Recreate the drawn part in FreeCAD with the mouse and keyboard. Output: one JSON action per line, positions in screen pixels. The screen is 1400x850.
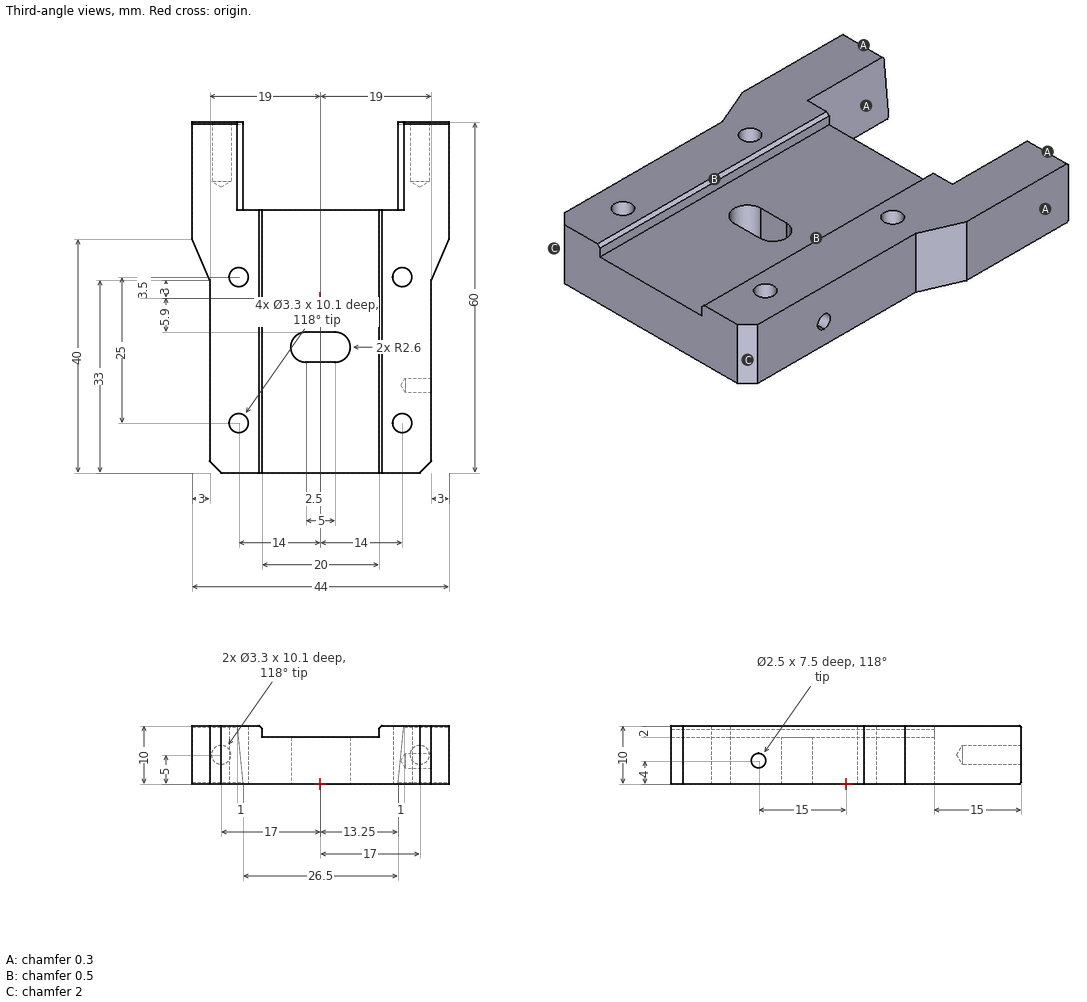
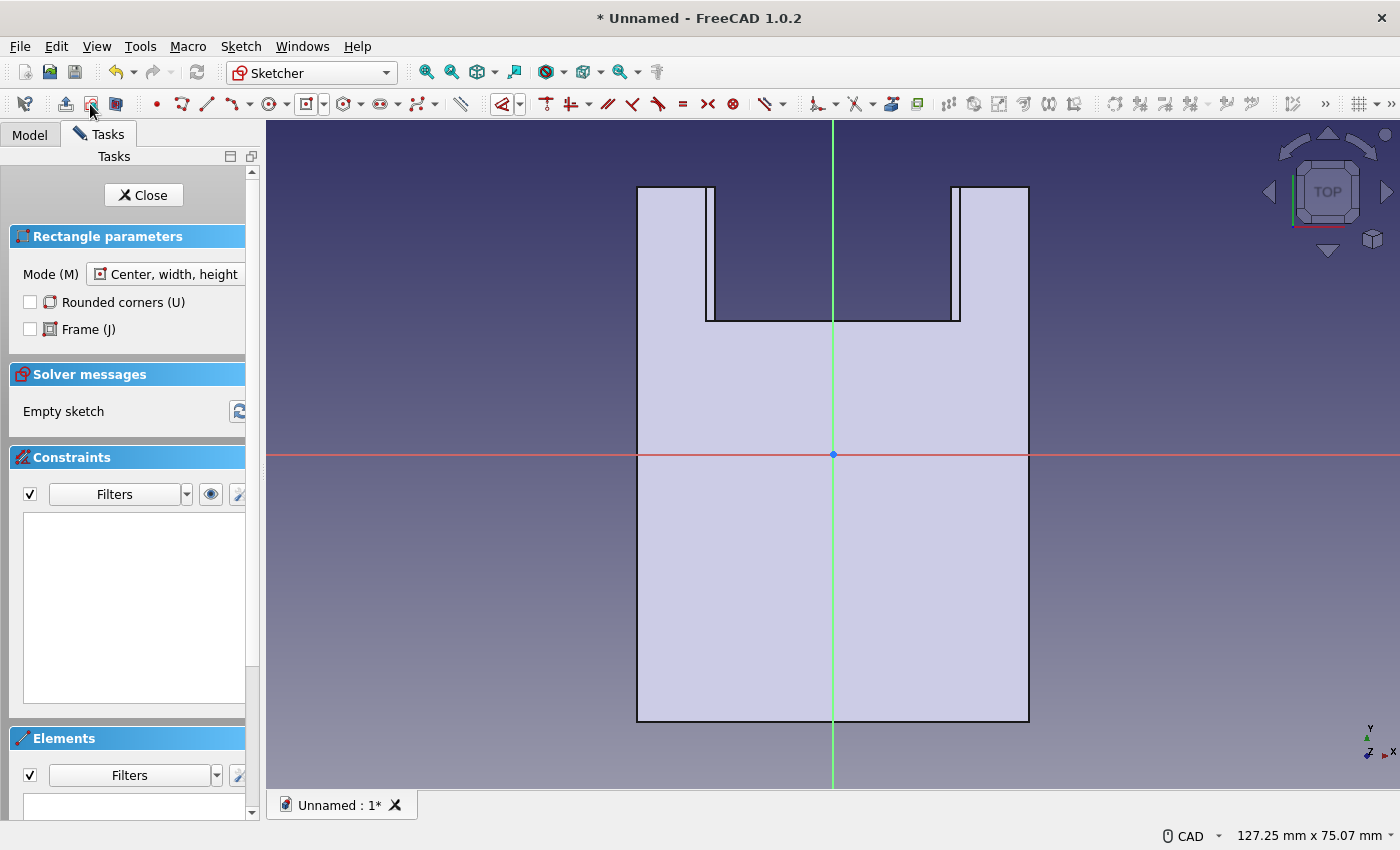
{"action": "left_click", "coordinate": [833, 454]}
{"action": "left_click", "coordinate": [922, 187]}
{"action": "key", "text": "Escape"}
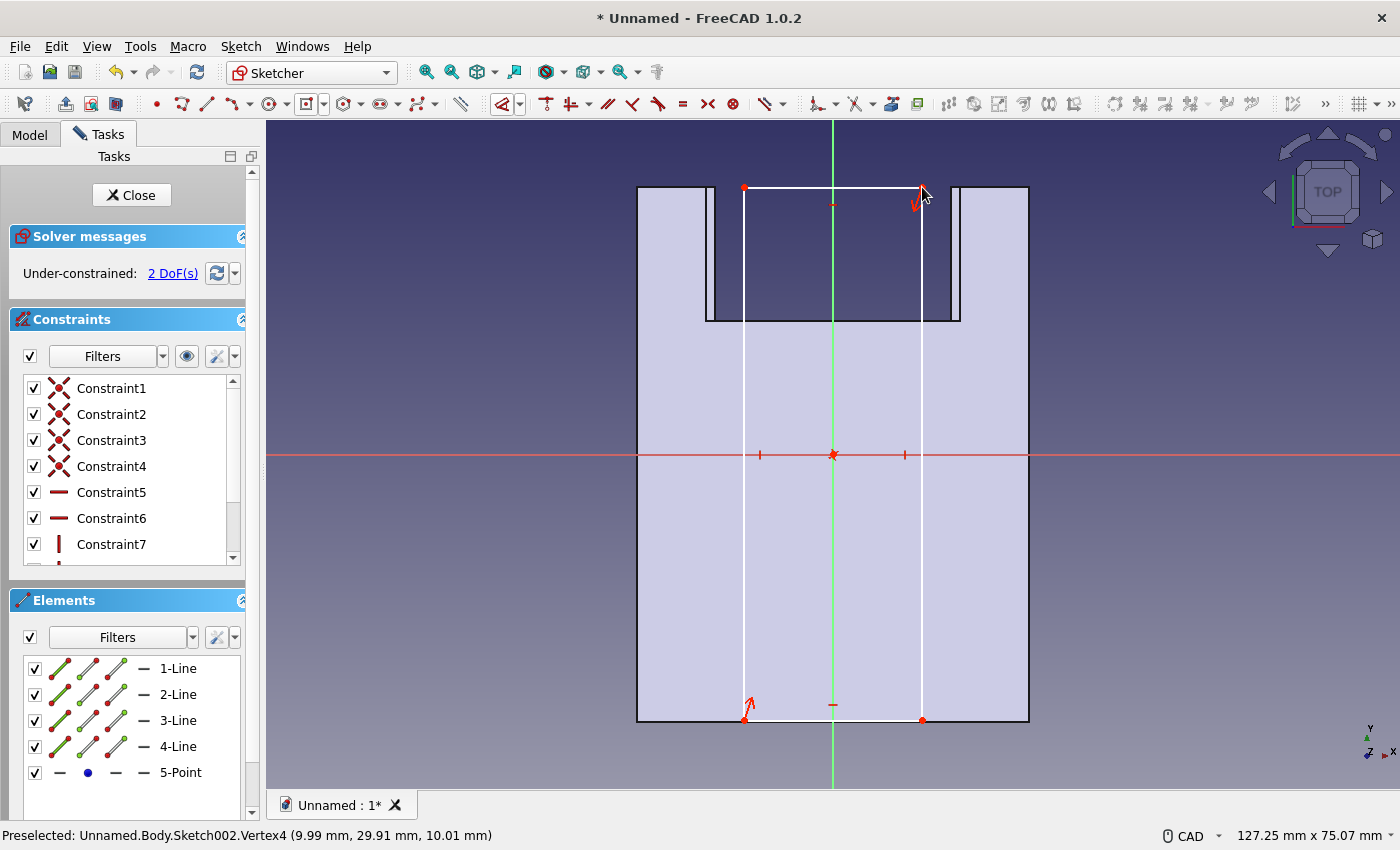
{"action": "left_click", "coordinate": [797, 721]}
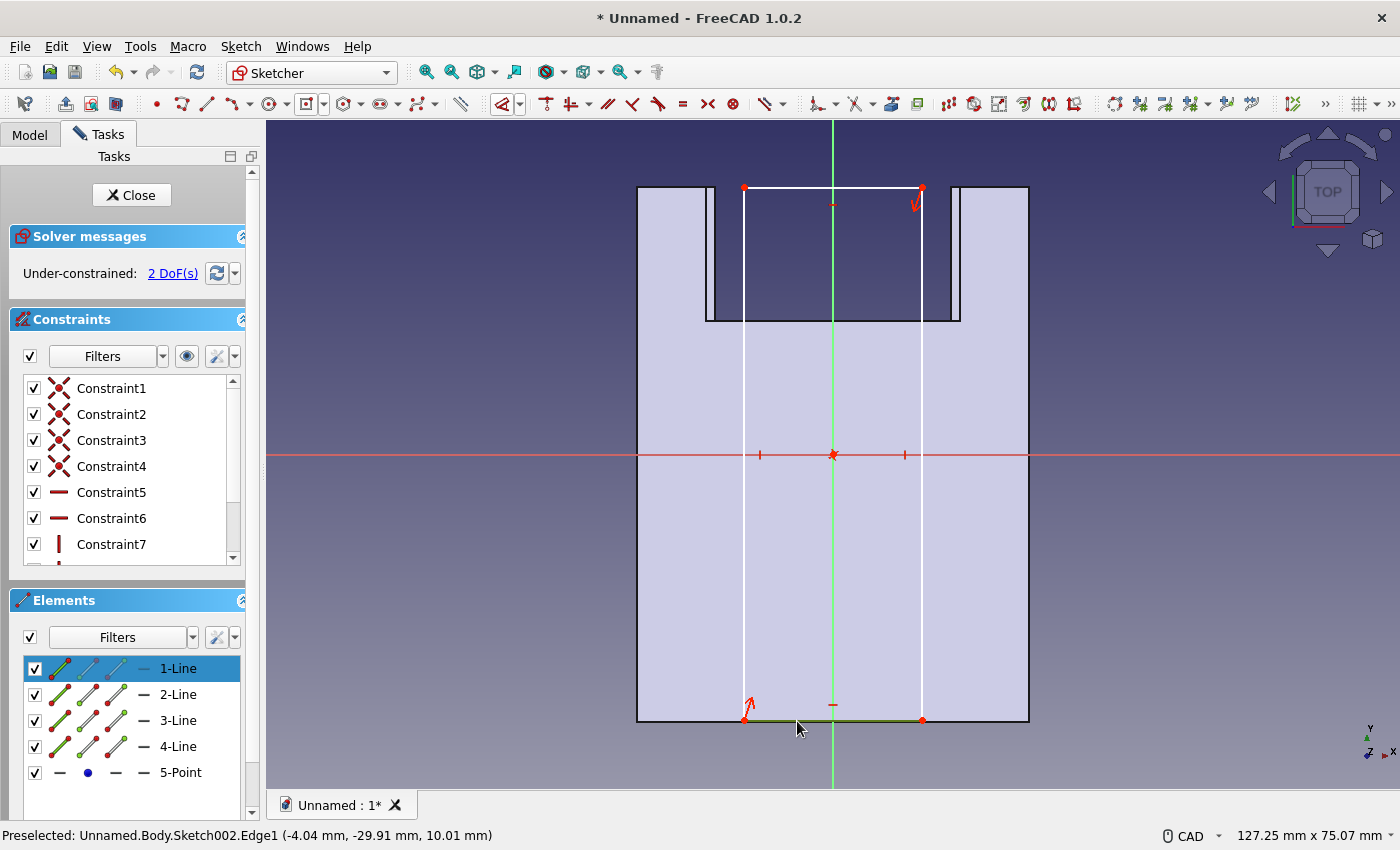
{"action": "key", "text": "l"}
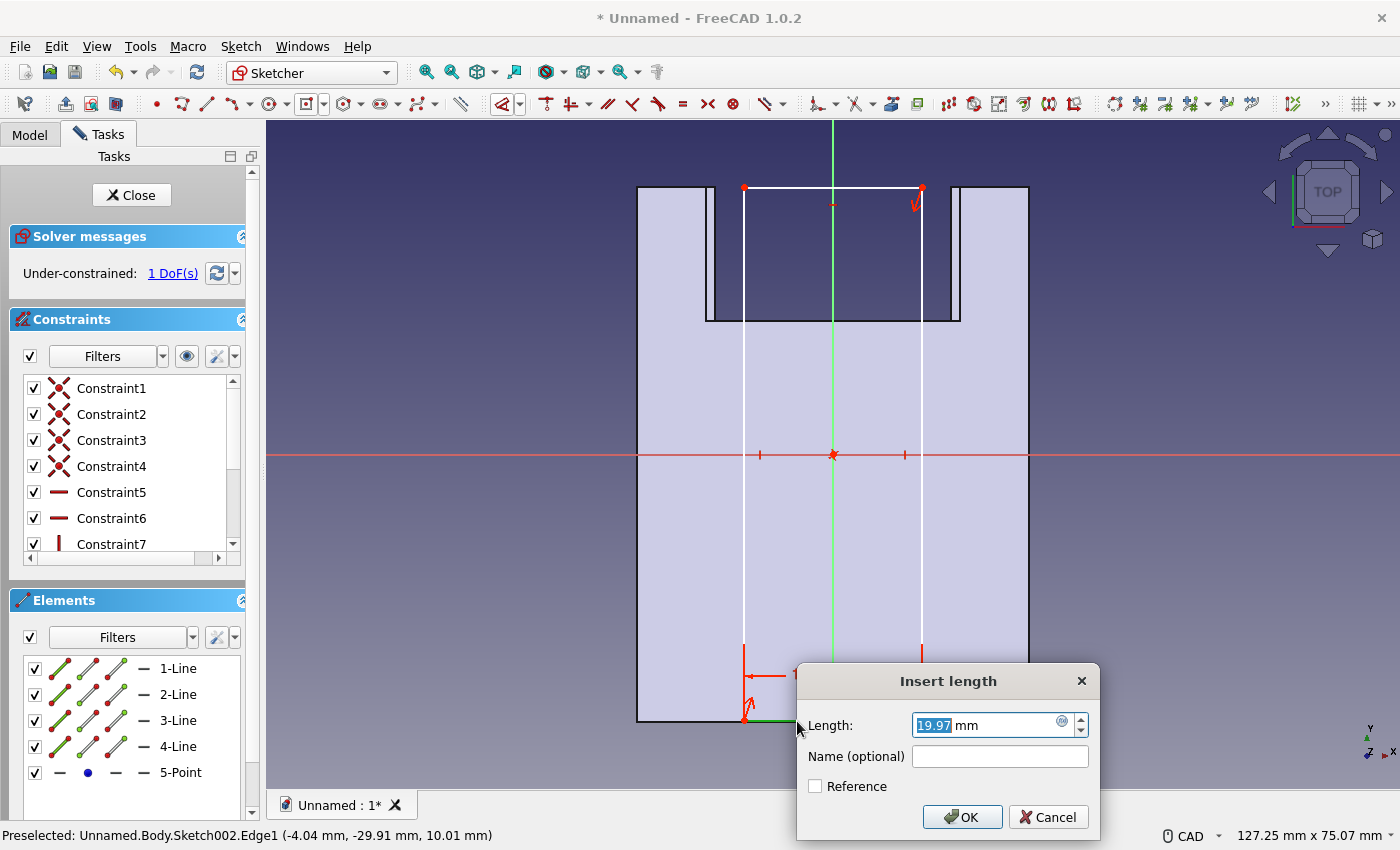
{"action": "type", "text": "20"}
{"action": "key", "text": "Return"}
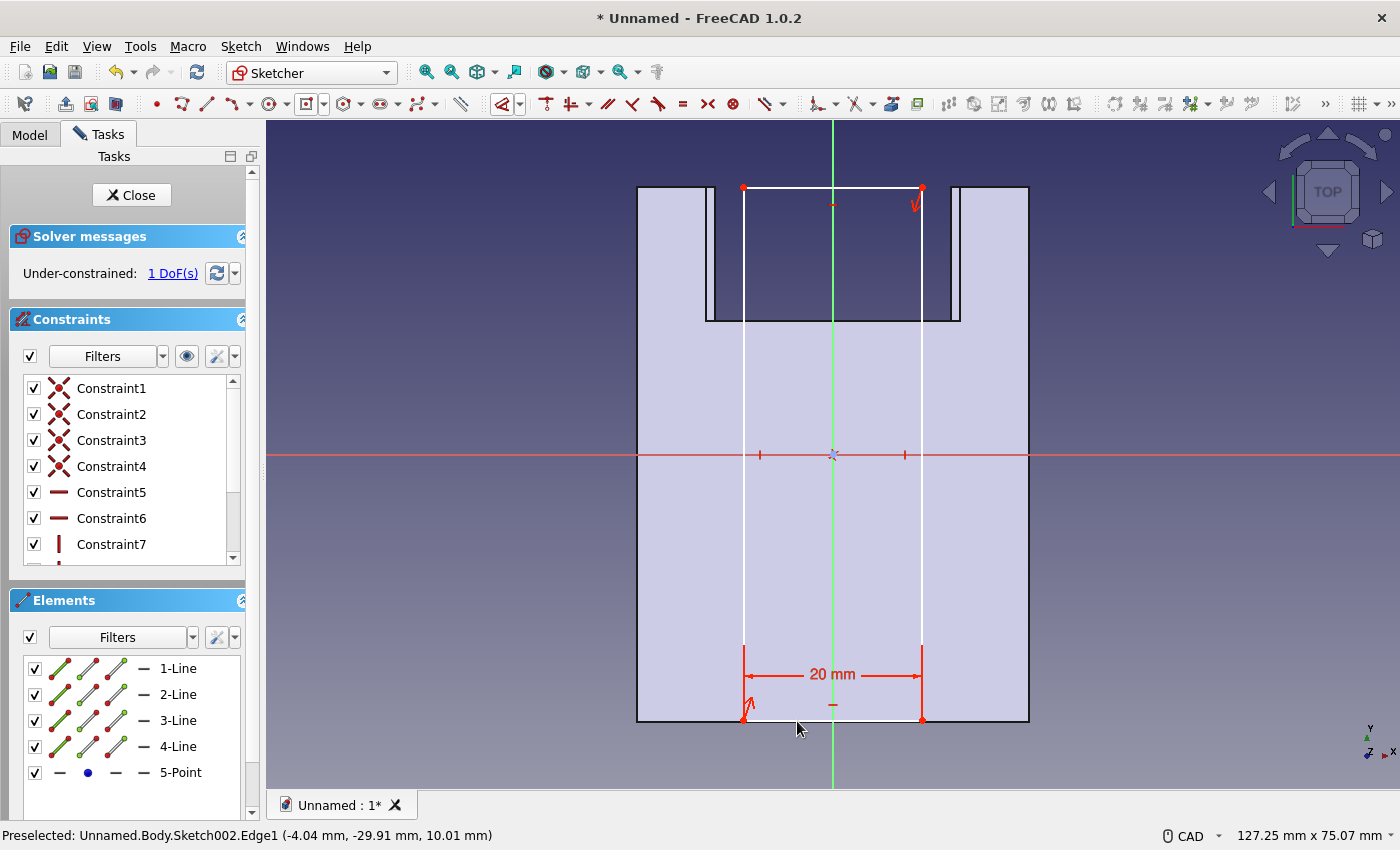
{"action": "left_click", "coordinate": [922, 561]}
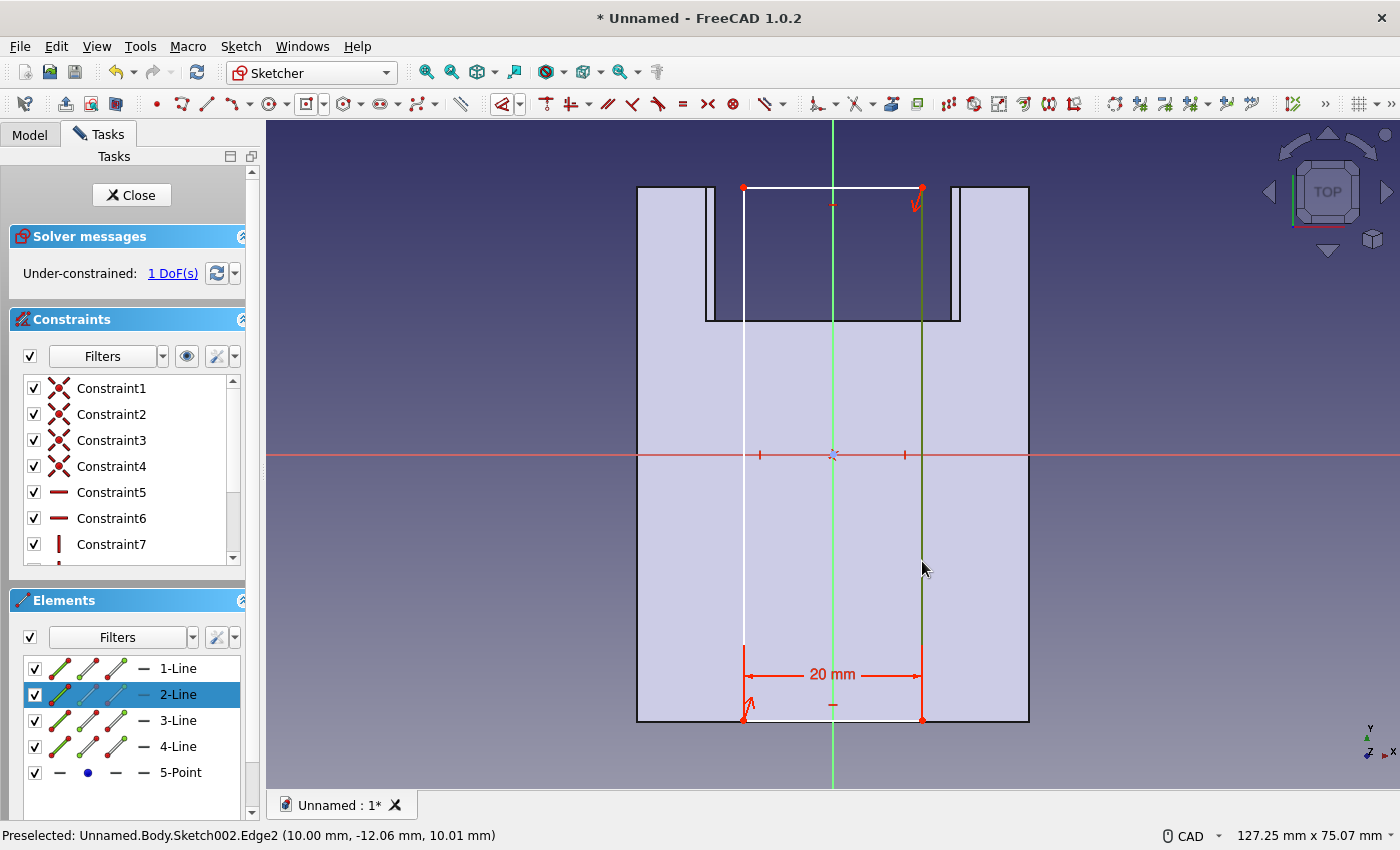
{"action": "key", "text": "i"}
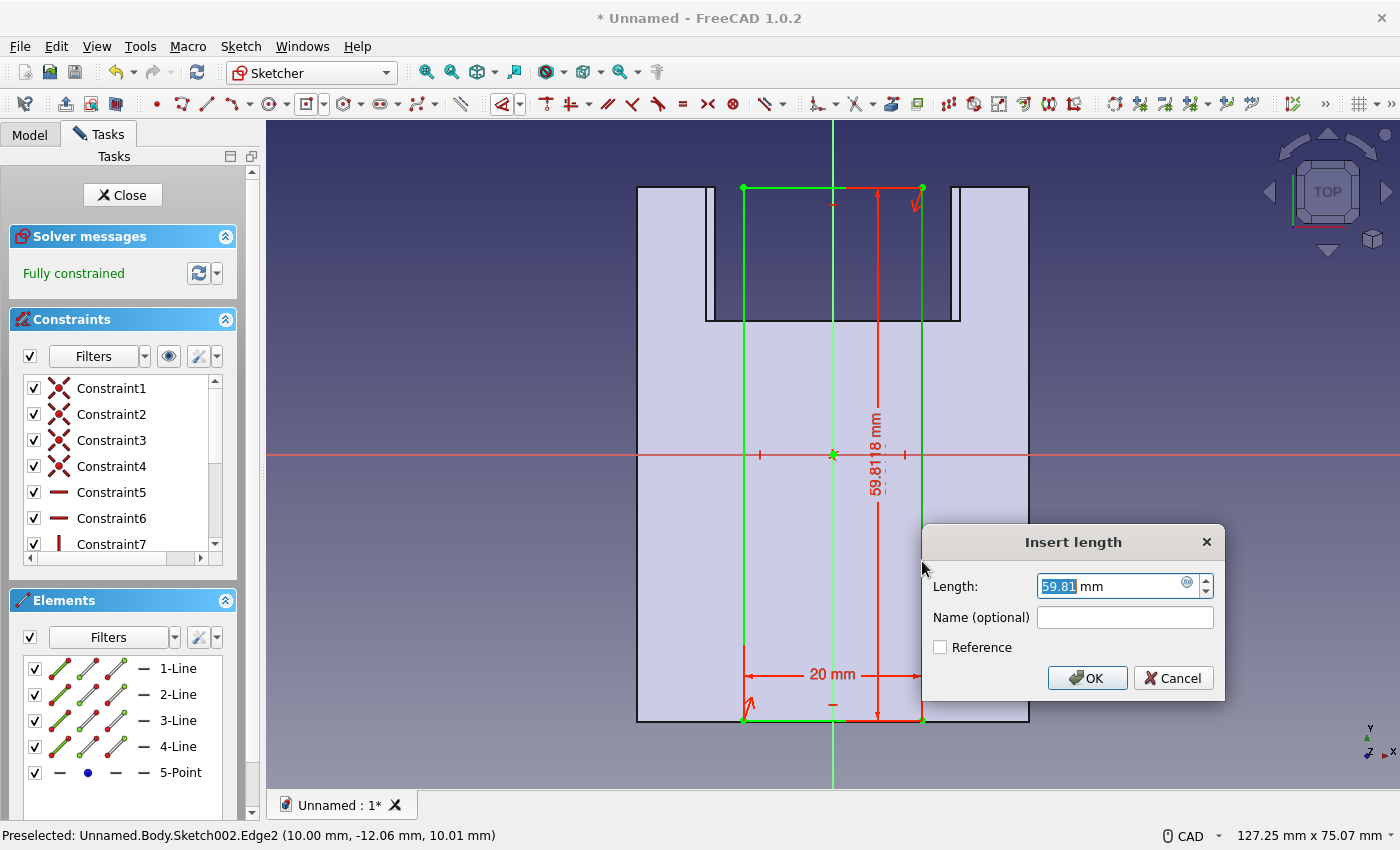
{"action": "type", "text": "60"}
{"action": "key", "text": "Return"}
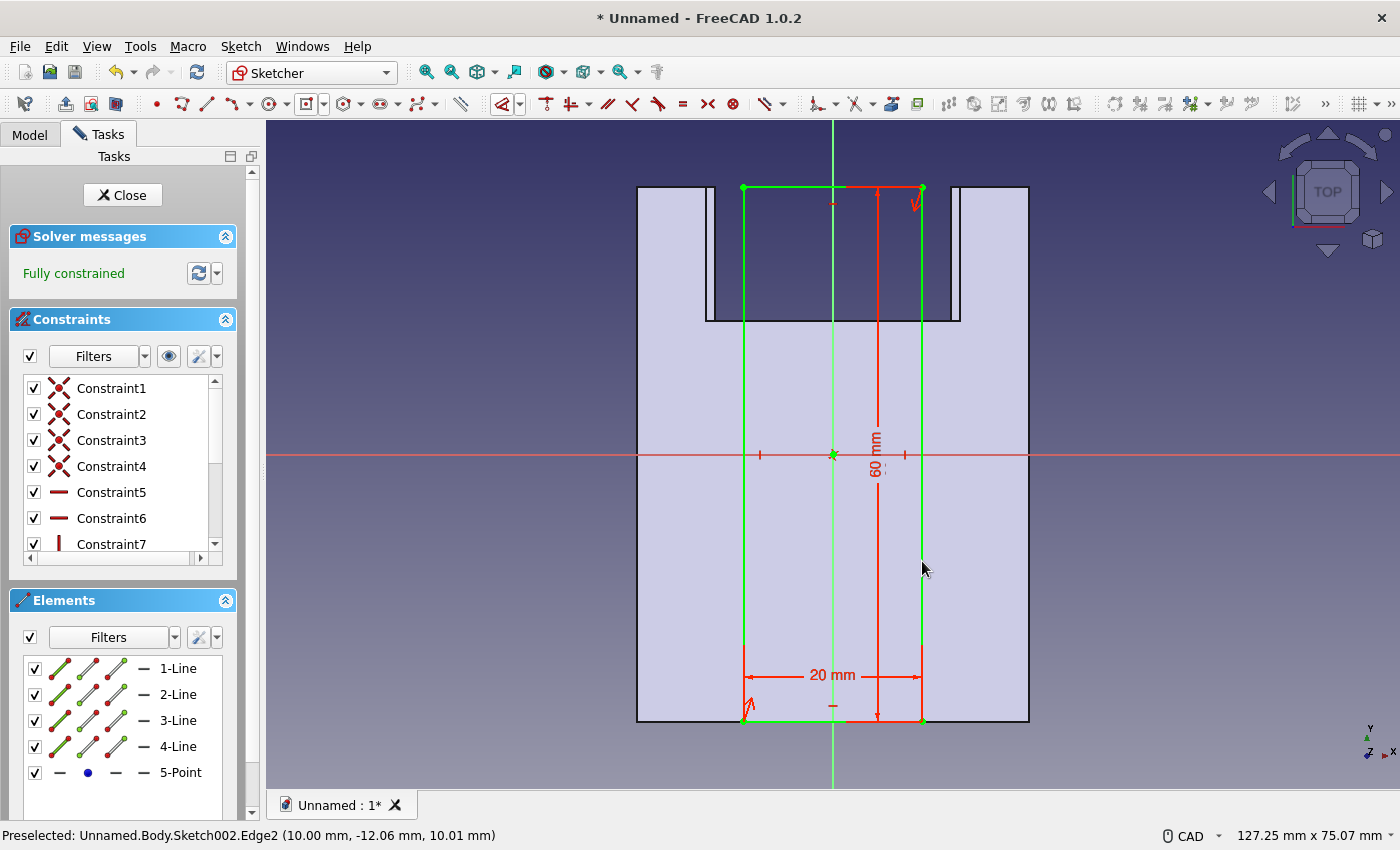
{"action": "left_click", "coordinate": [123, 195]}